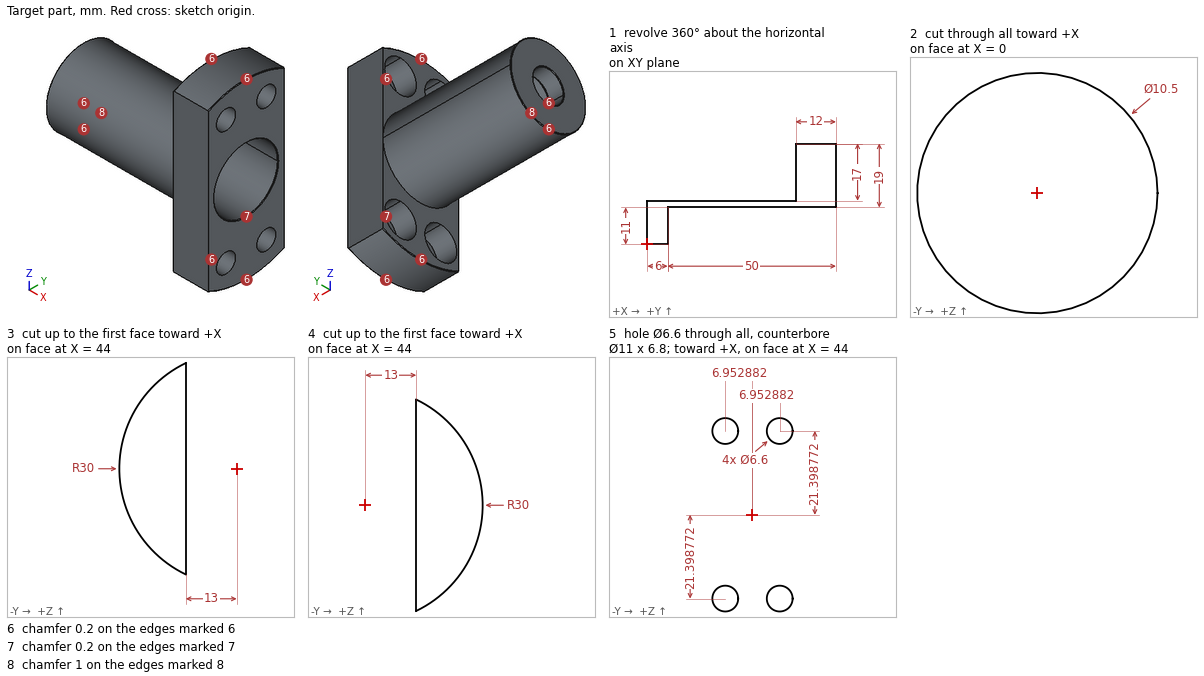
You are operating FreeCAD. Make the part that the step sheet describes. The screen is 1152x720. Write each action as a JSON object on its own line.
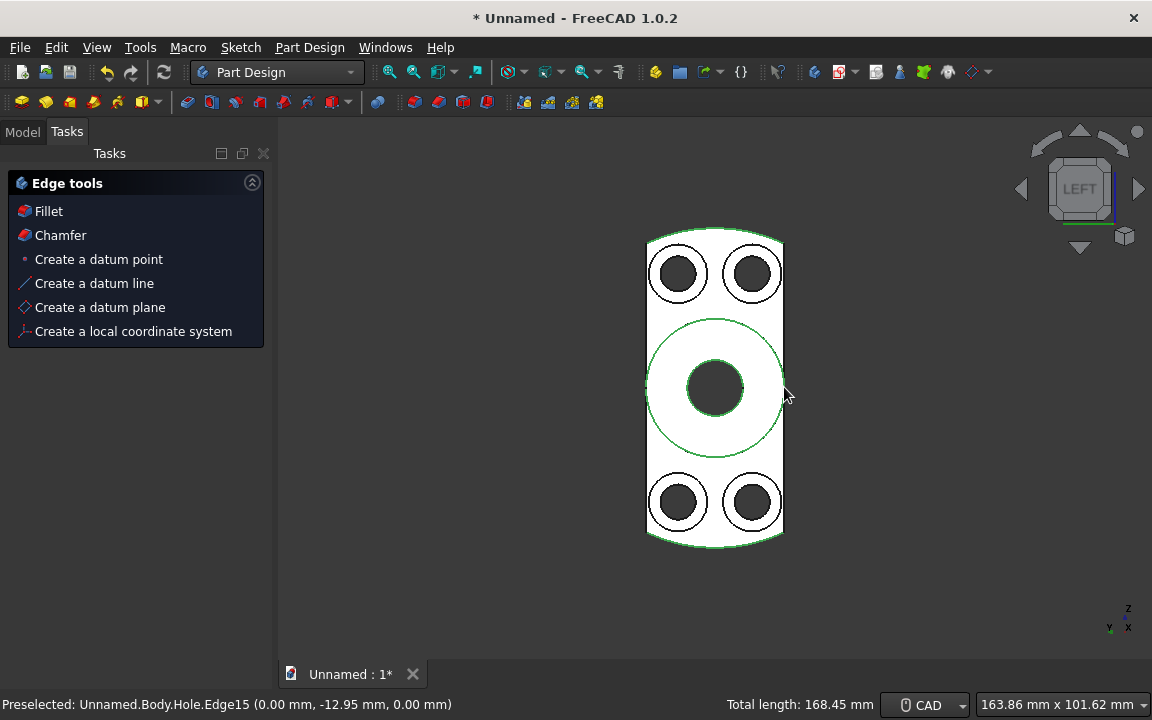
{"action": "key", "text": "0"}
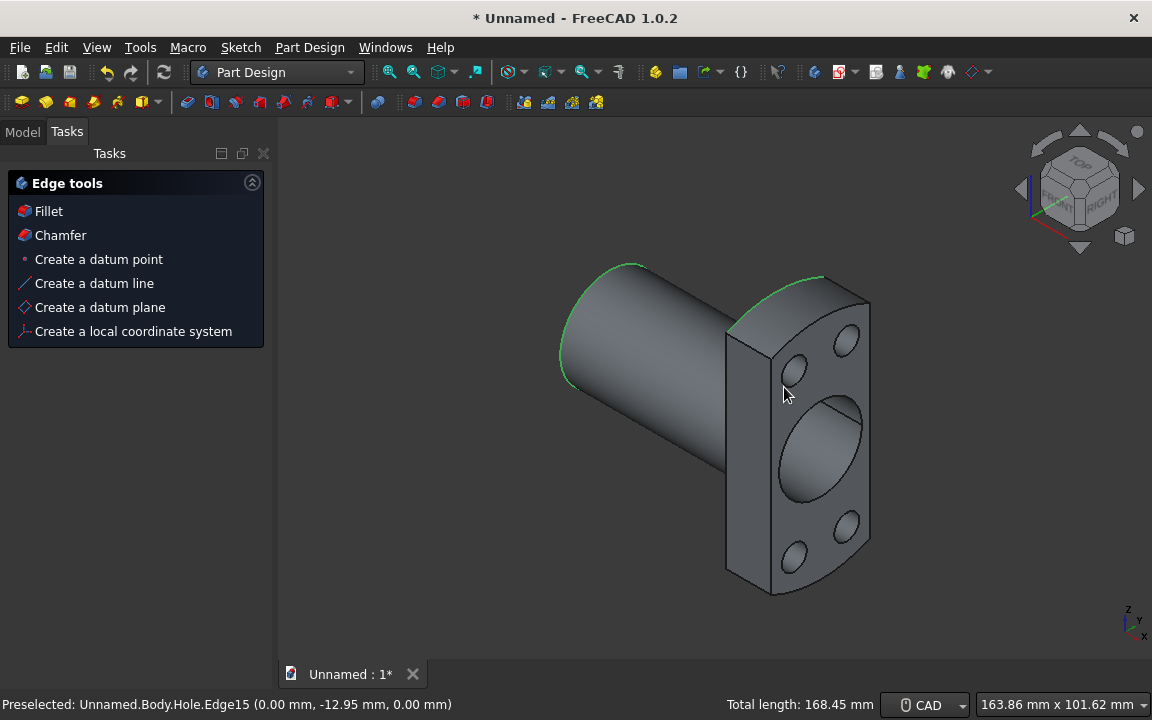
{"action": "left_click", "coordinate": [820, 317], "text": "ctrl"}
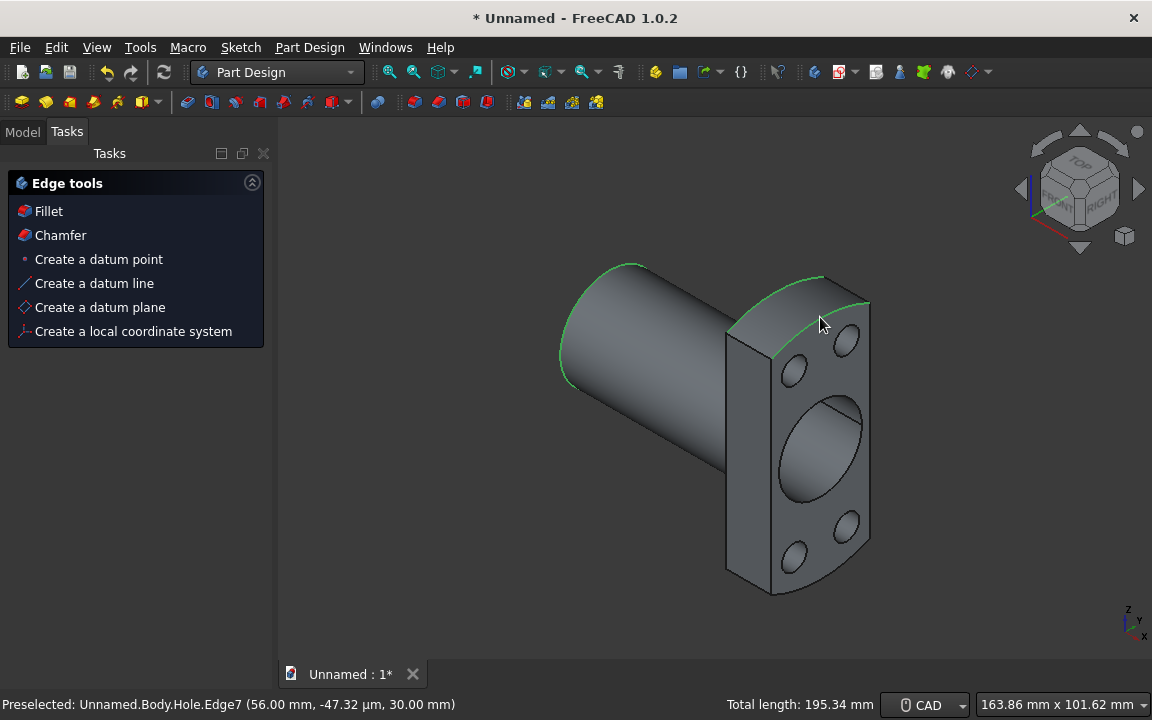
{"action": "key", "text": "2"}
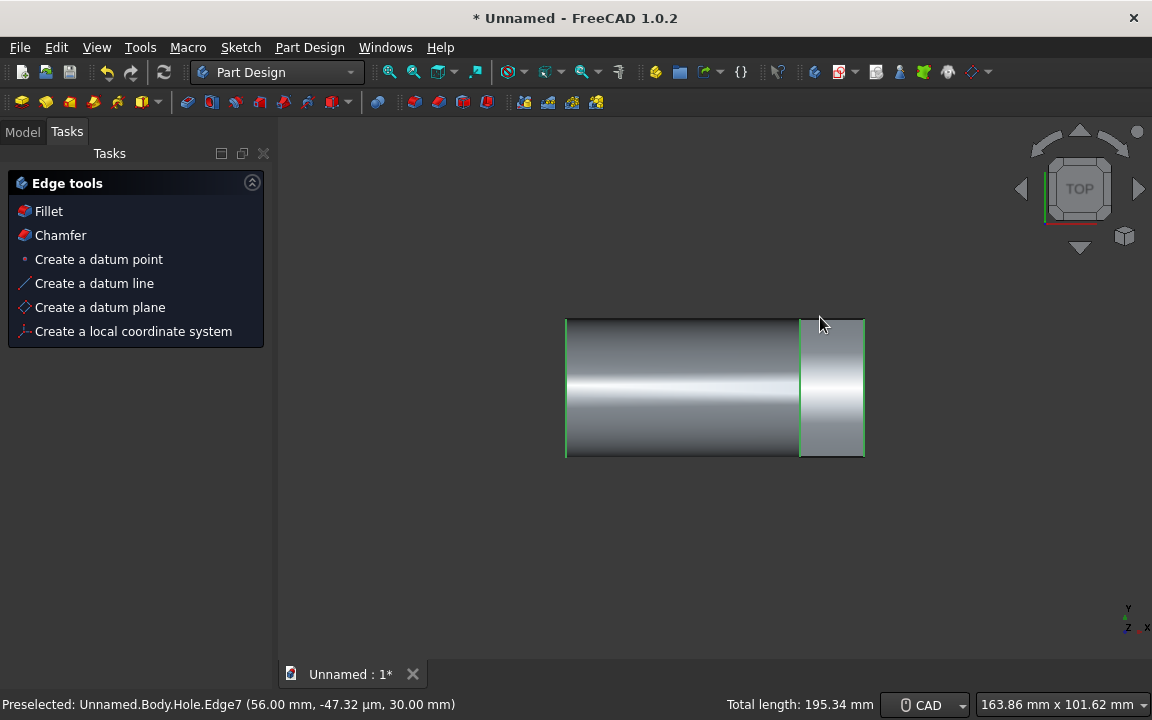
{"action": "key", "text": "v f"}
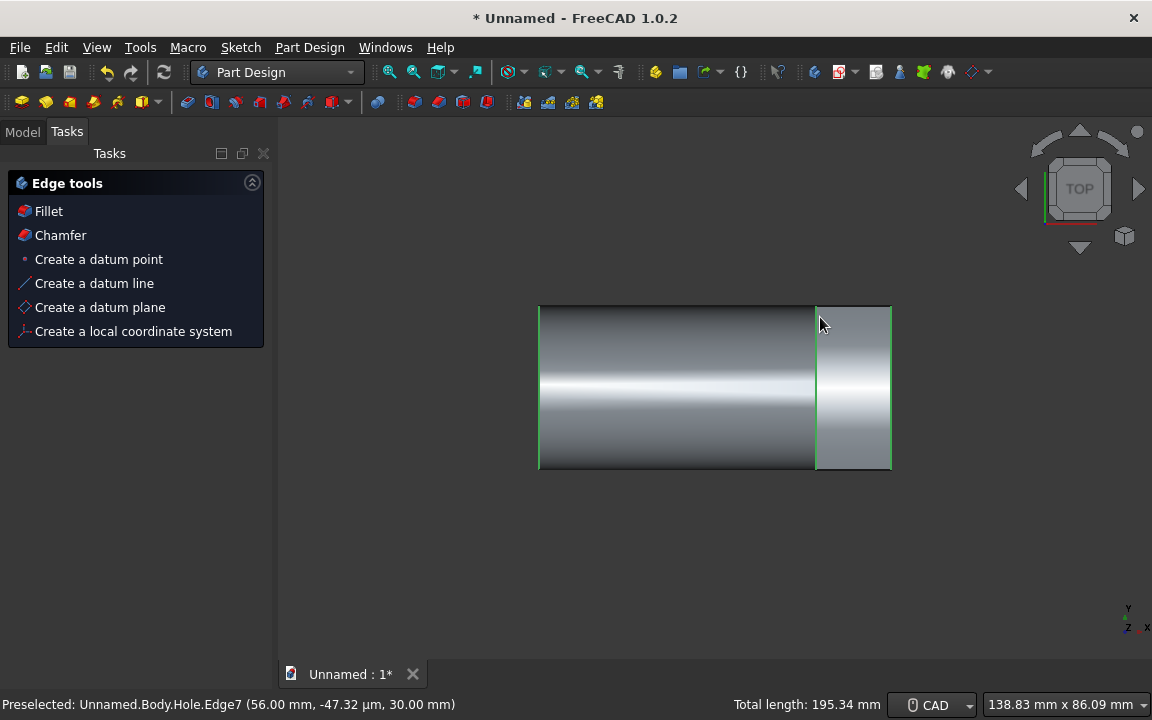
{"action": "key", "text": "1"}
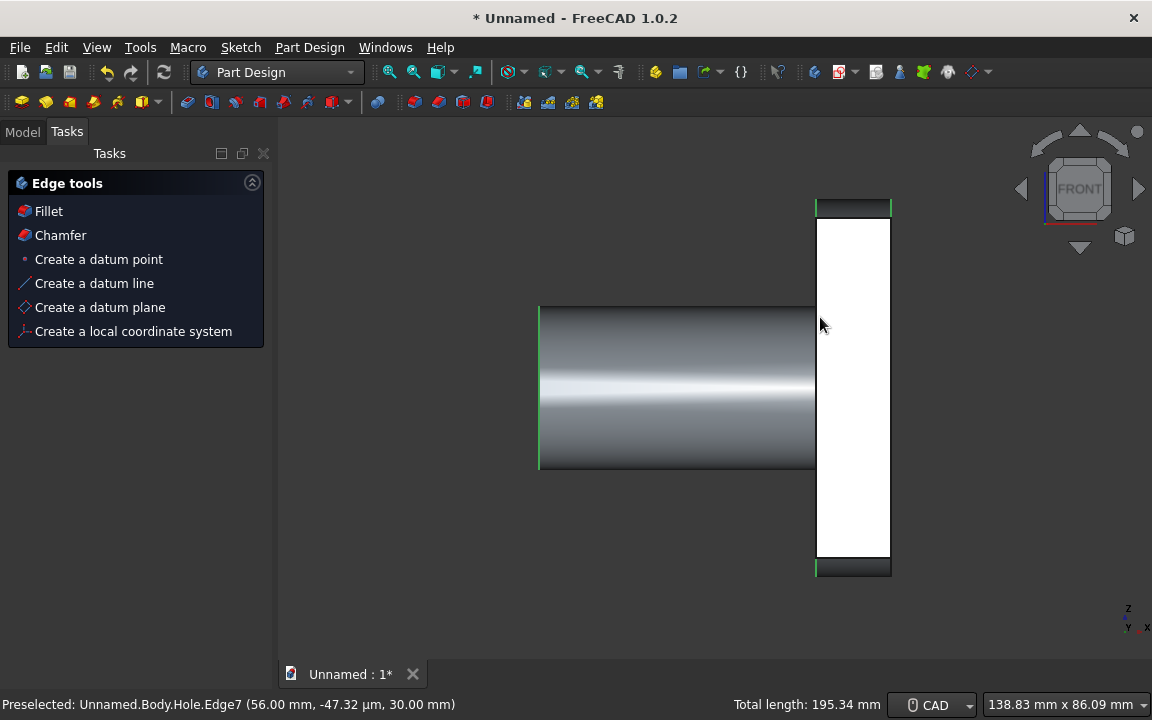
{"action": "left_click", "coordinate": [891, 575], "text": "ctrl"}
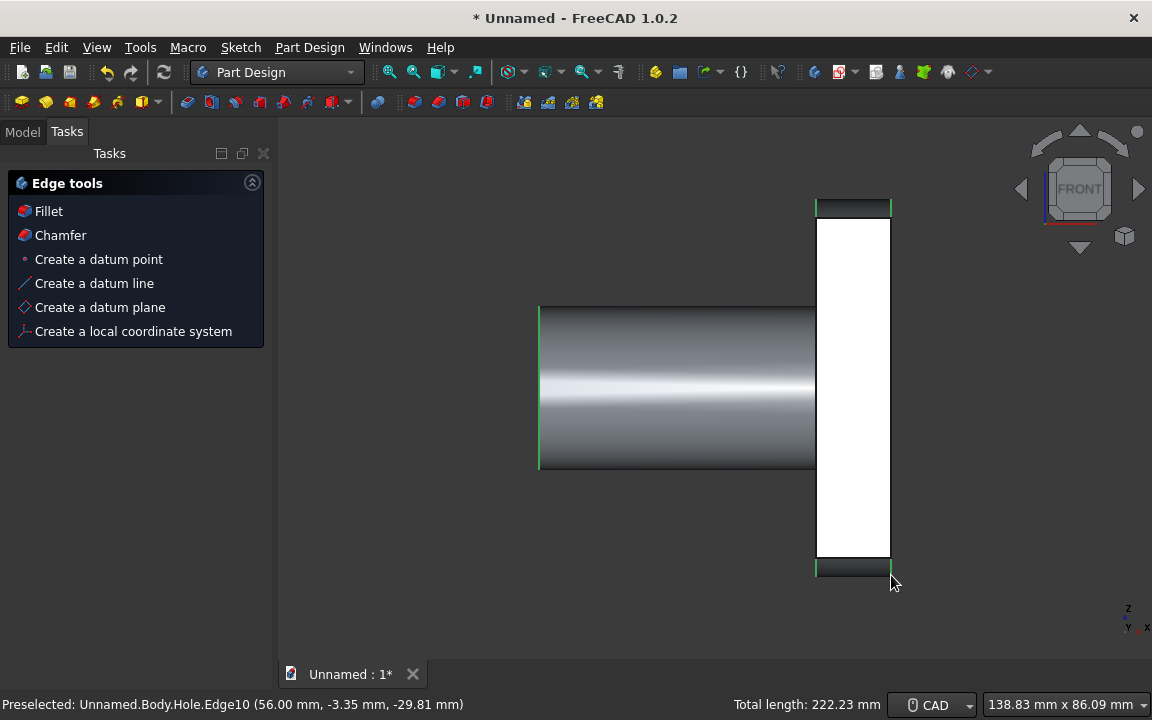
{"action": "left_click", "coordinate": [440, 102]}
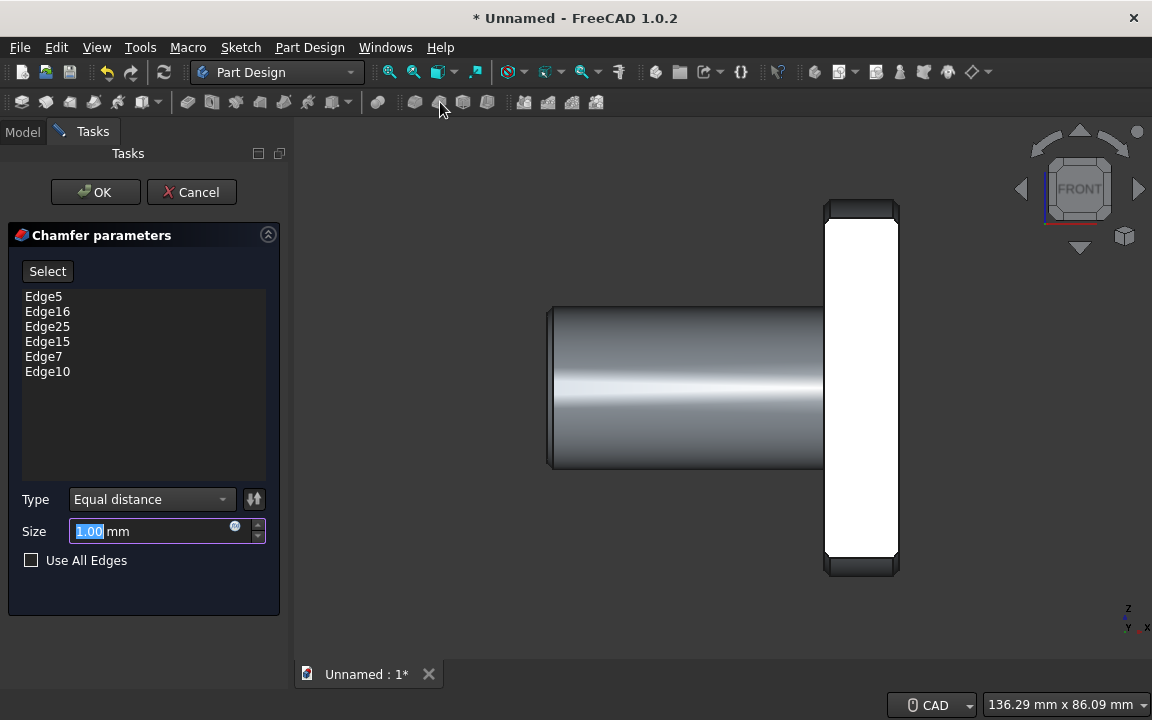
{"action": "type", "text": "0.2"}
{"action": "key", "text": "Tab"}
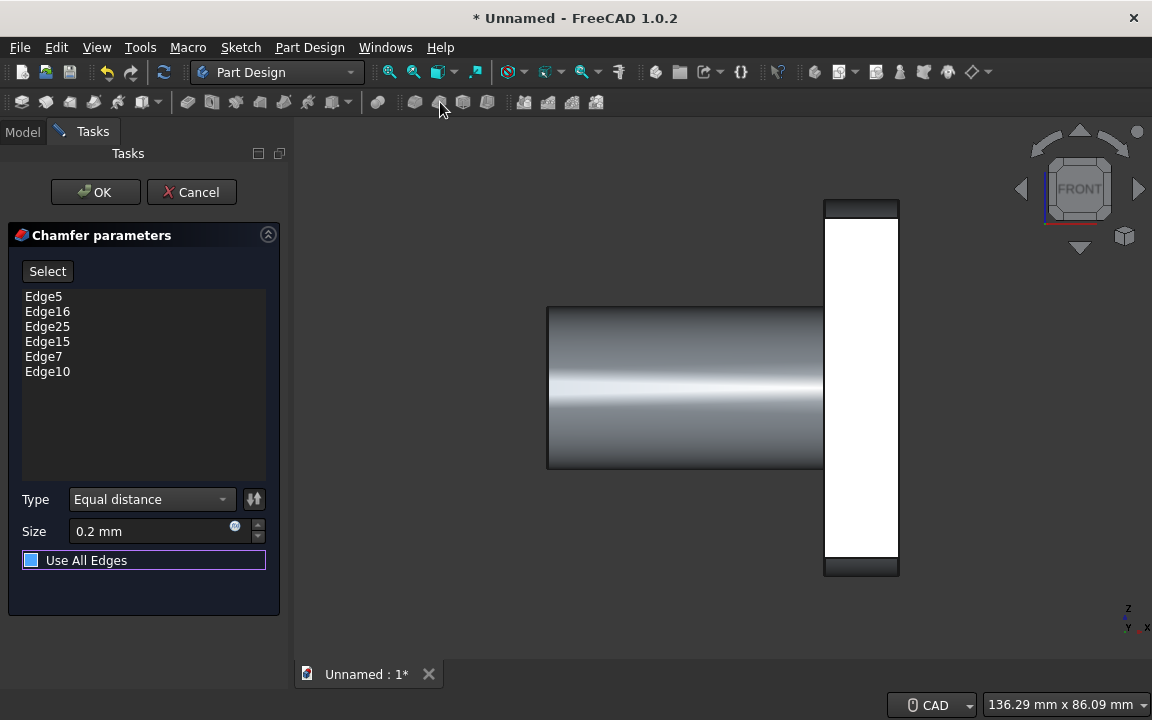
{"action": "left_click", "coordinate": [96, 192]}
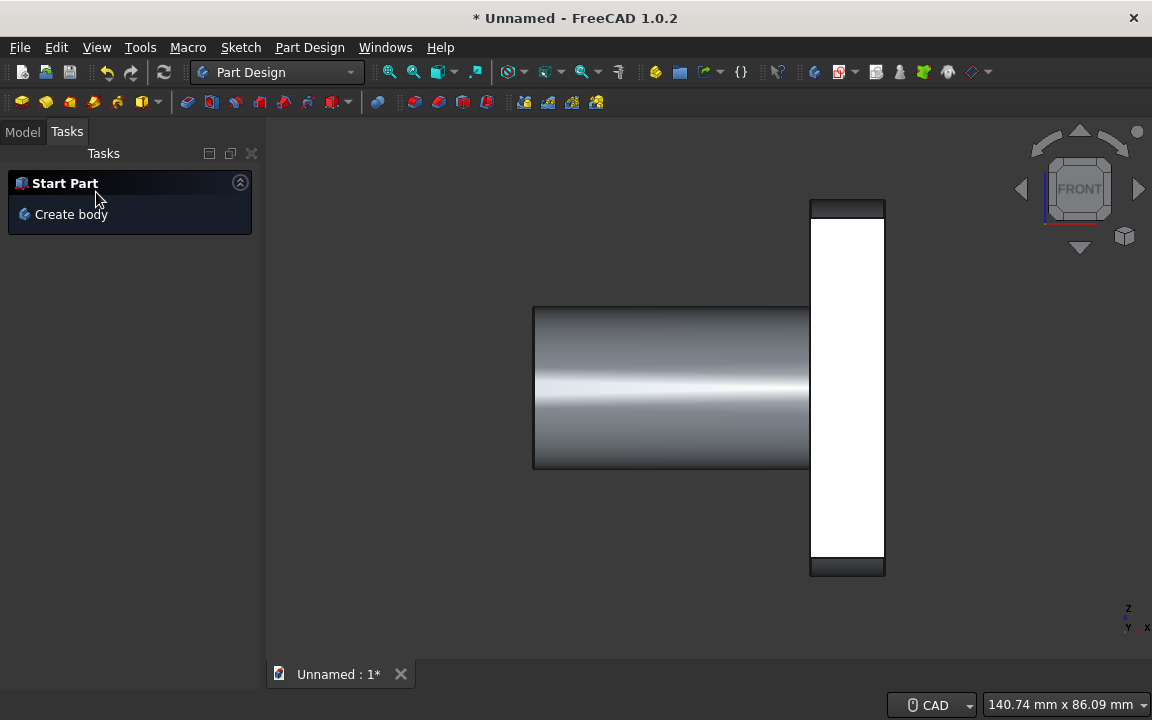
{"action": "key", "text": "0"}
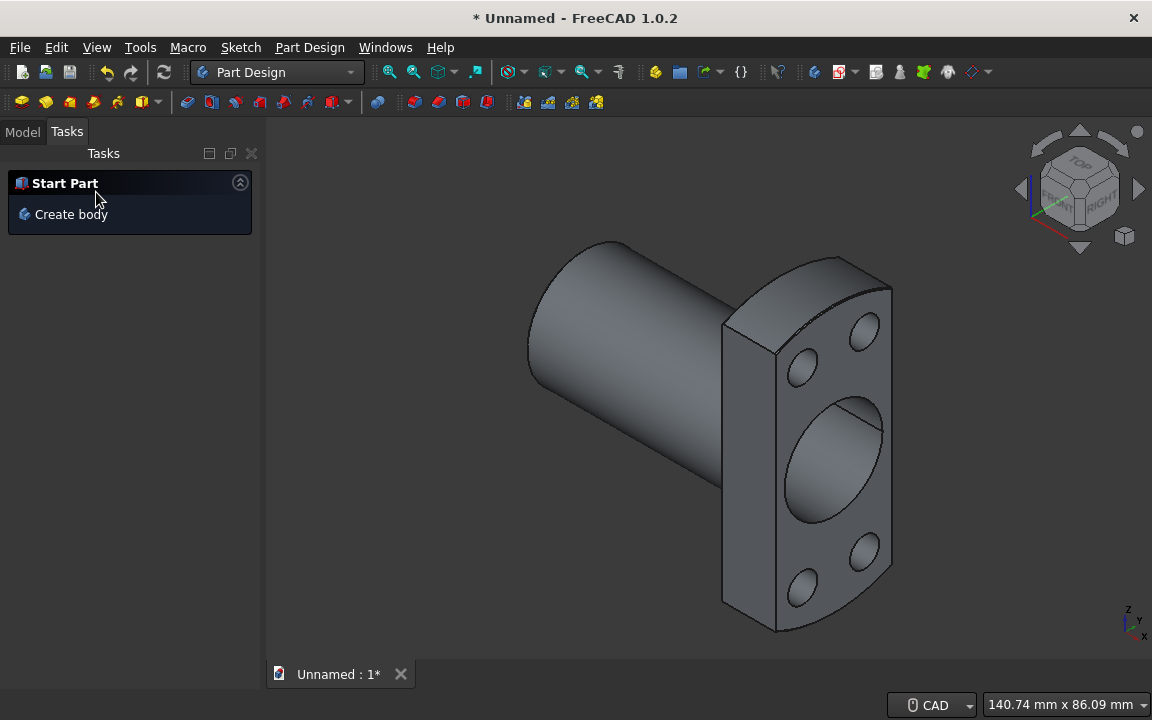
{"action": "left_click", "coordinate": [819, 521]}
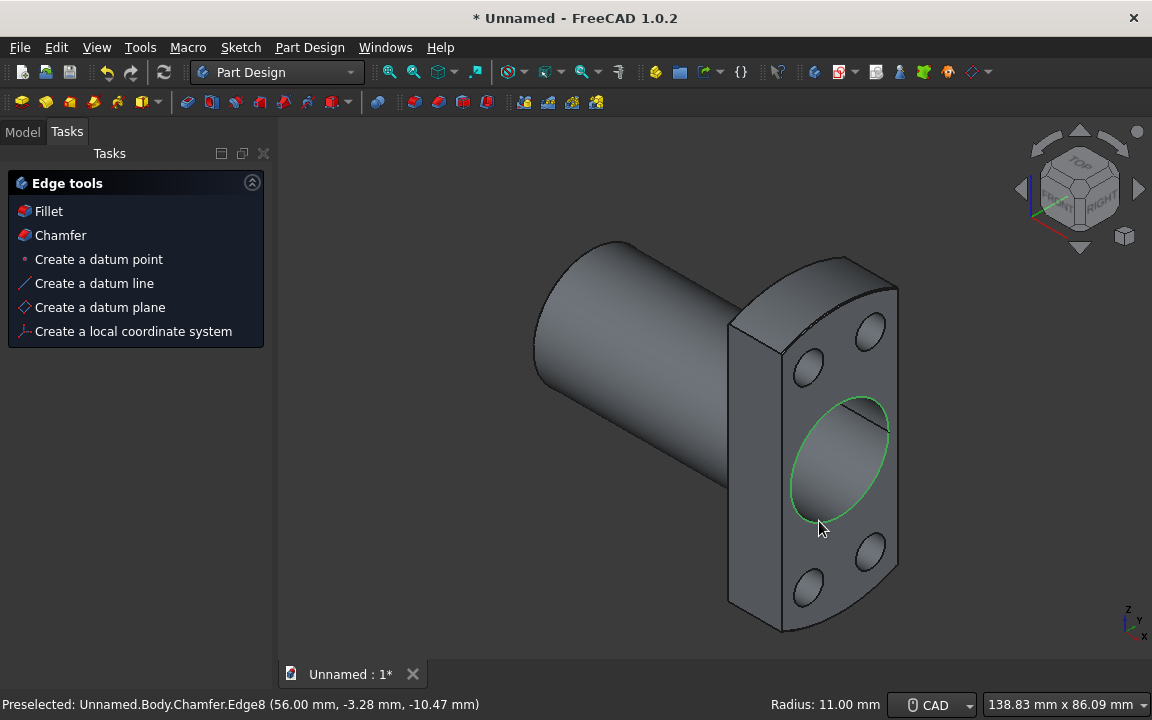
{"action": "left_click", "coordinate": [440, 102]}